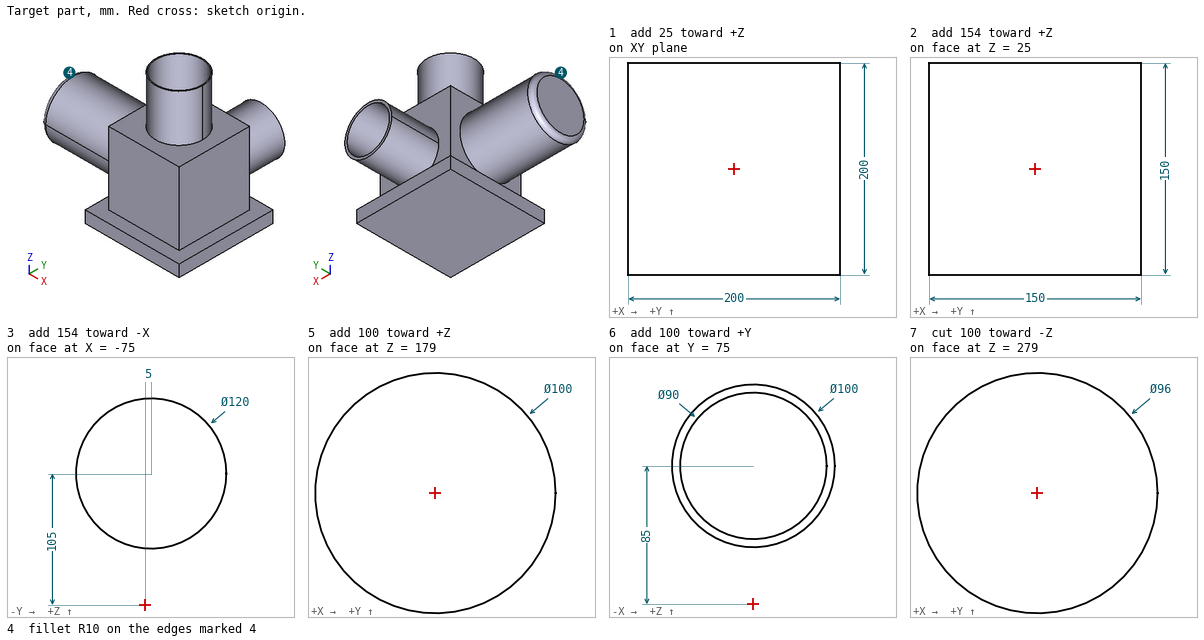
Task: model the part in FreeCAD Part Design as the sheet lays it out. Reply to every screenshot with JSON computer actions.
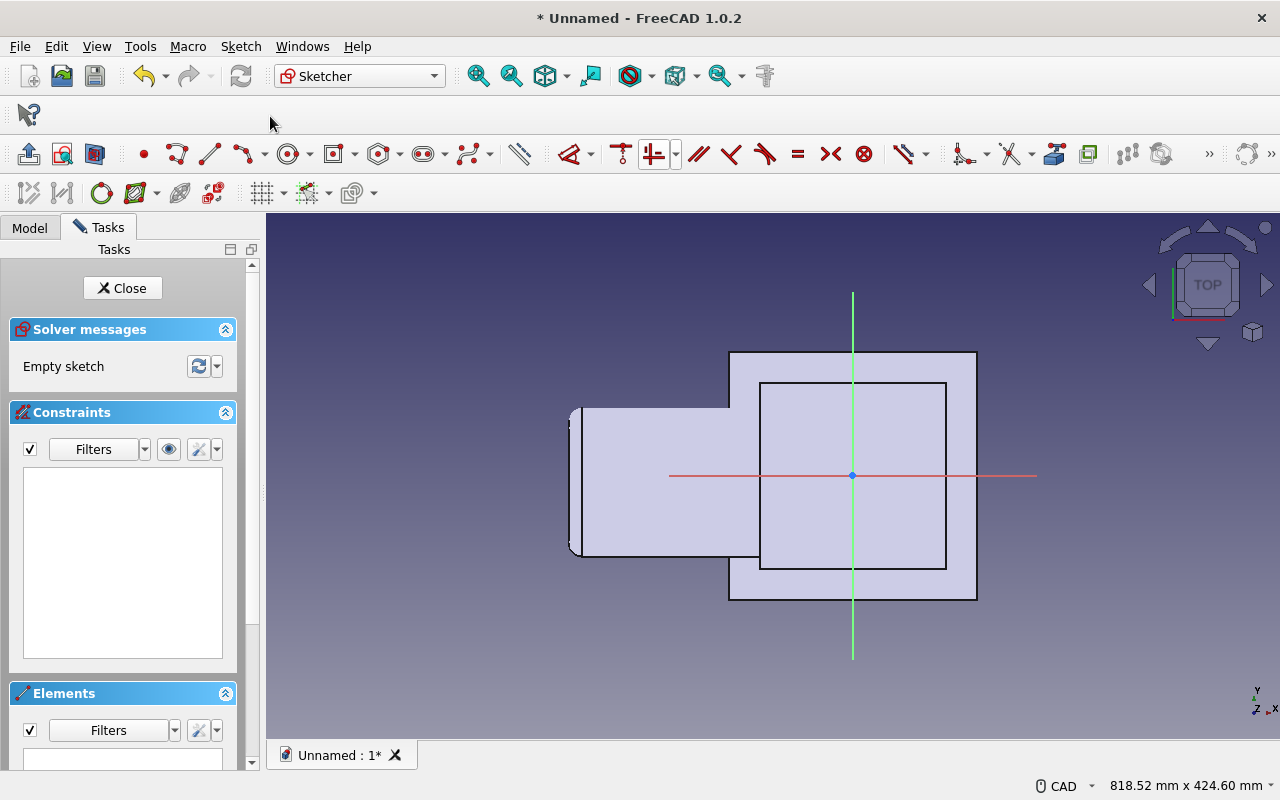
{"action": "scroll", "coordinate": [939, 476], "scroll_direction": "up", "scroll_amount": 5}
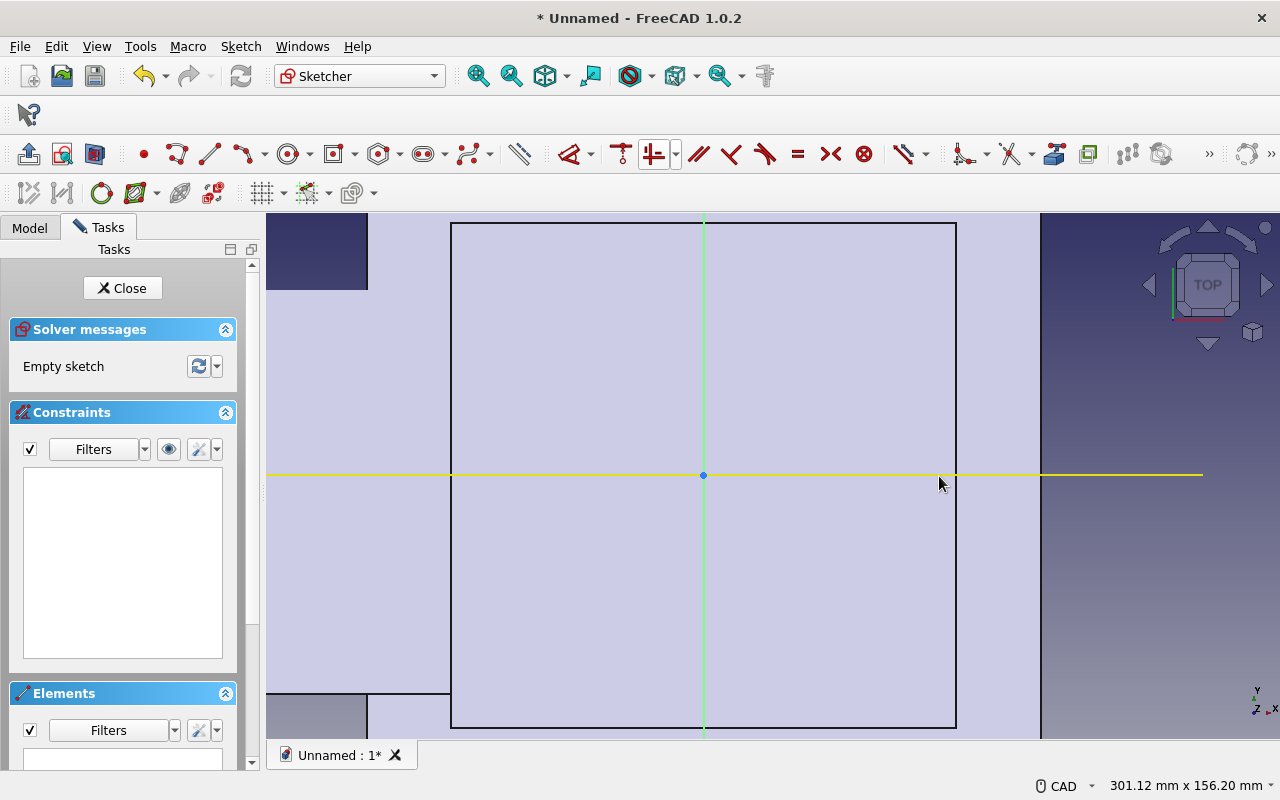
{"action": "left_click", "coordinate": [288, 154]}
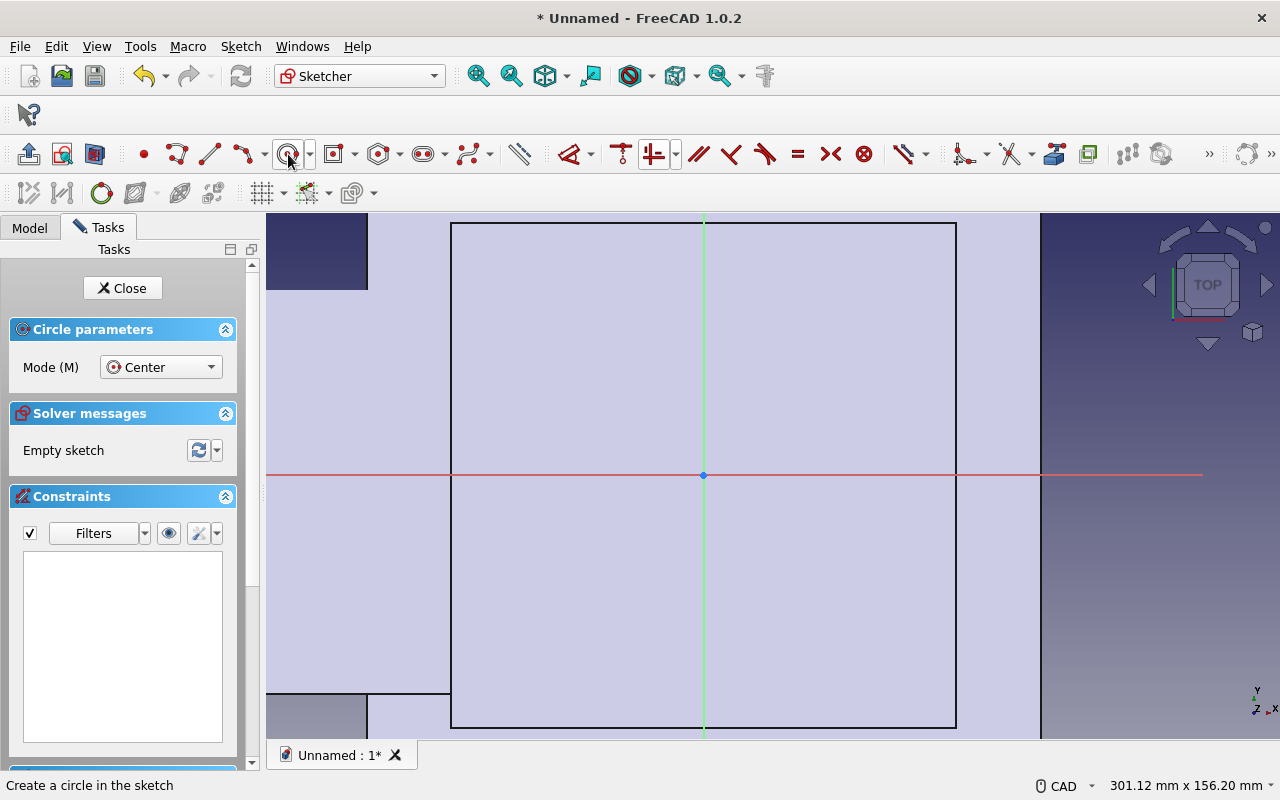
{"action": "left_click", "coordinate": [704, 475]}
{"action": "mouse_move", "coordinate": [823, 356]}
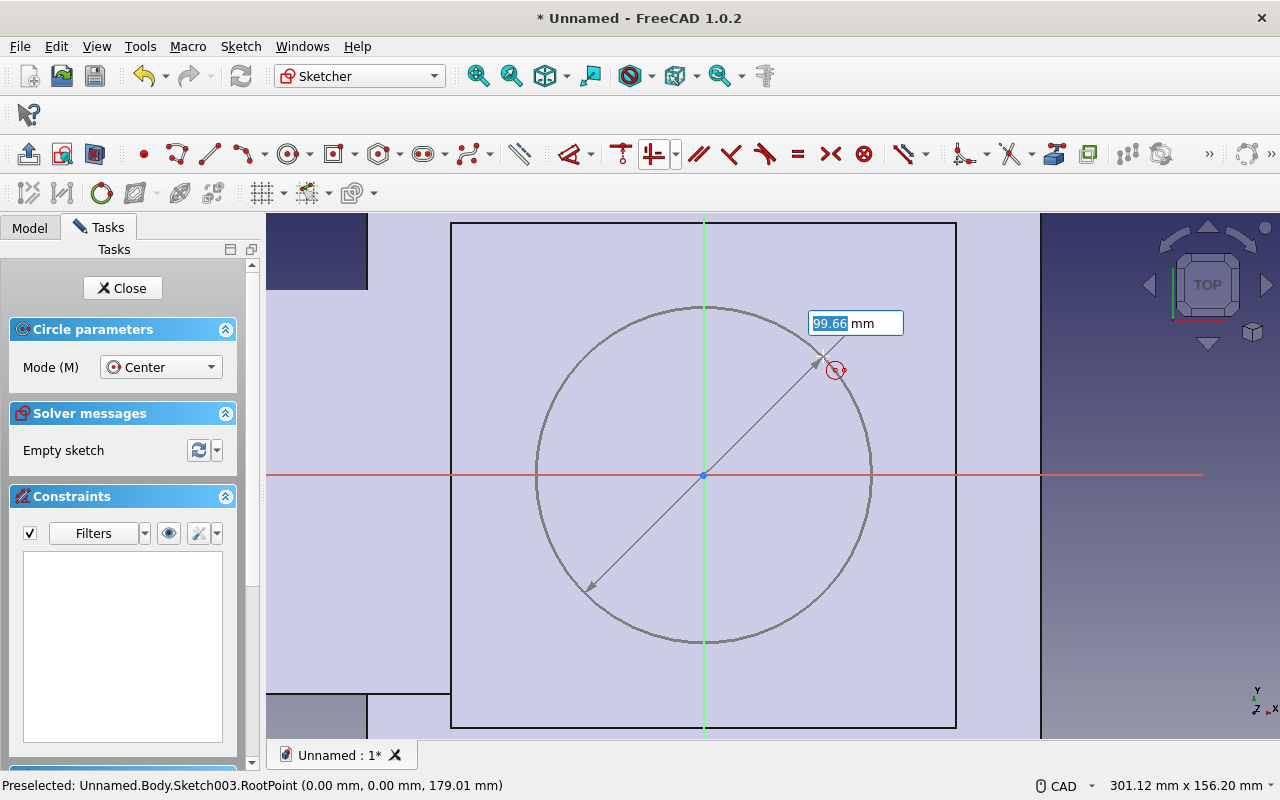
{"action": "type", "text": "100"}
{"action": "key", "text": "Return"}
{"action": "key", "text": "Escape"}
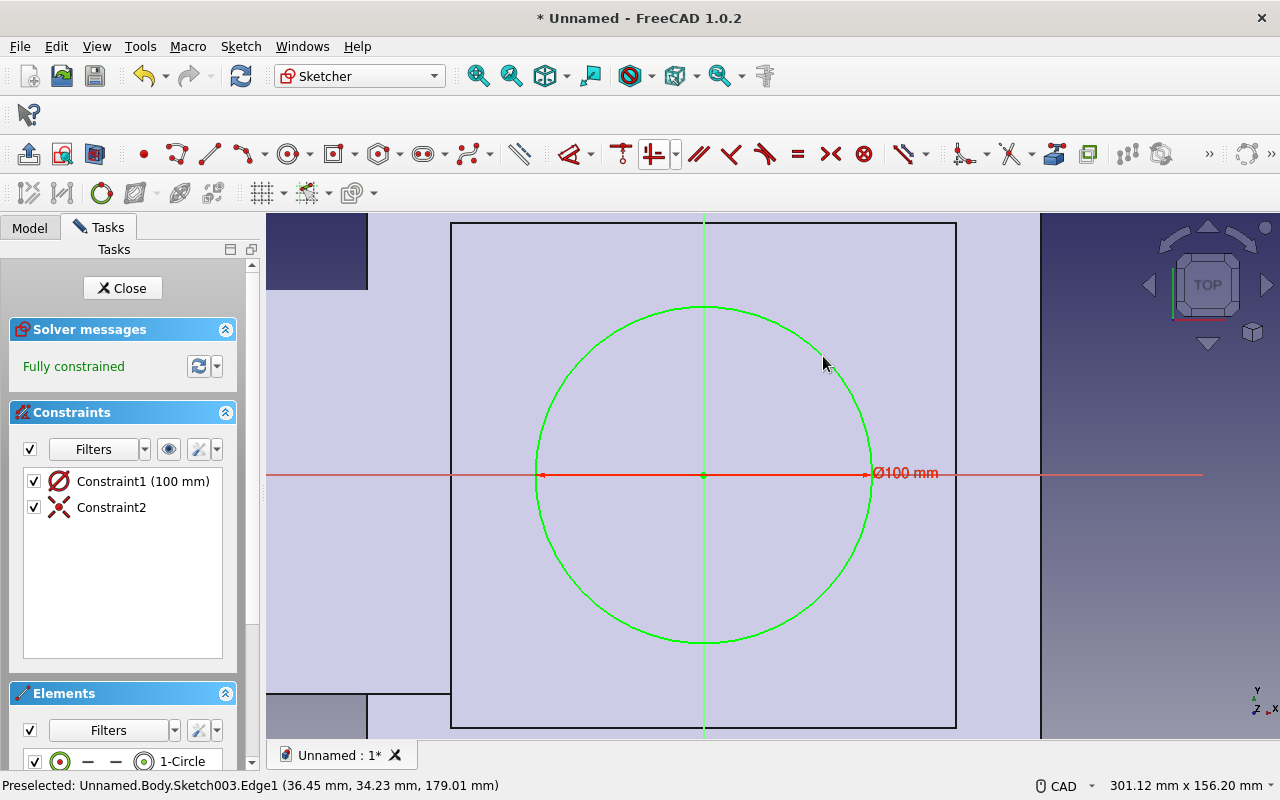
{"action": "left_click", "coordinate": [123, 288]}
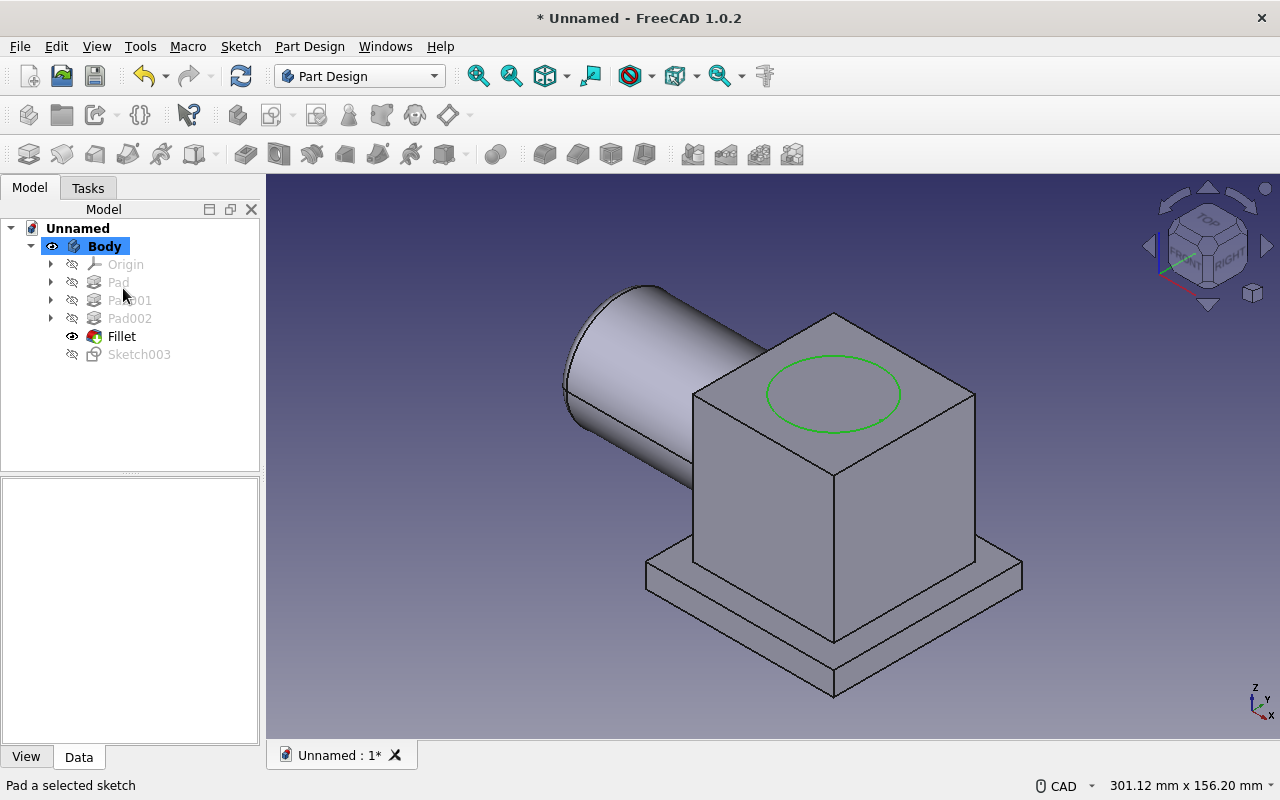
{"action": "left_click", "coordinate": [29, 154]}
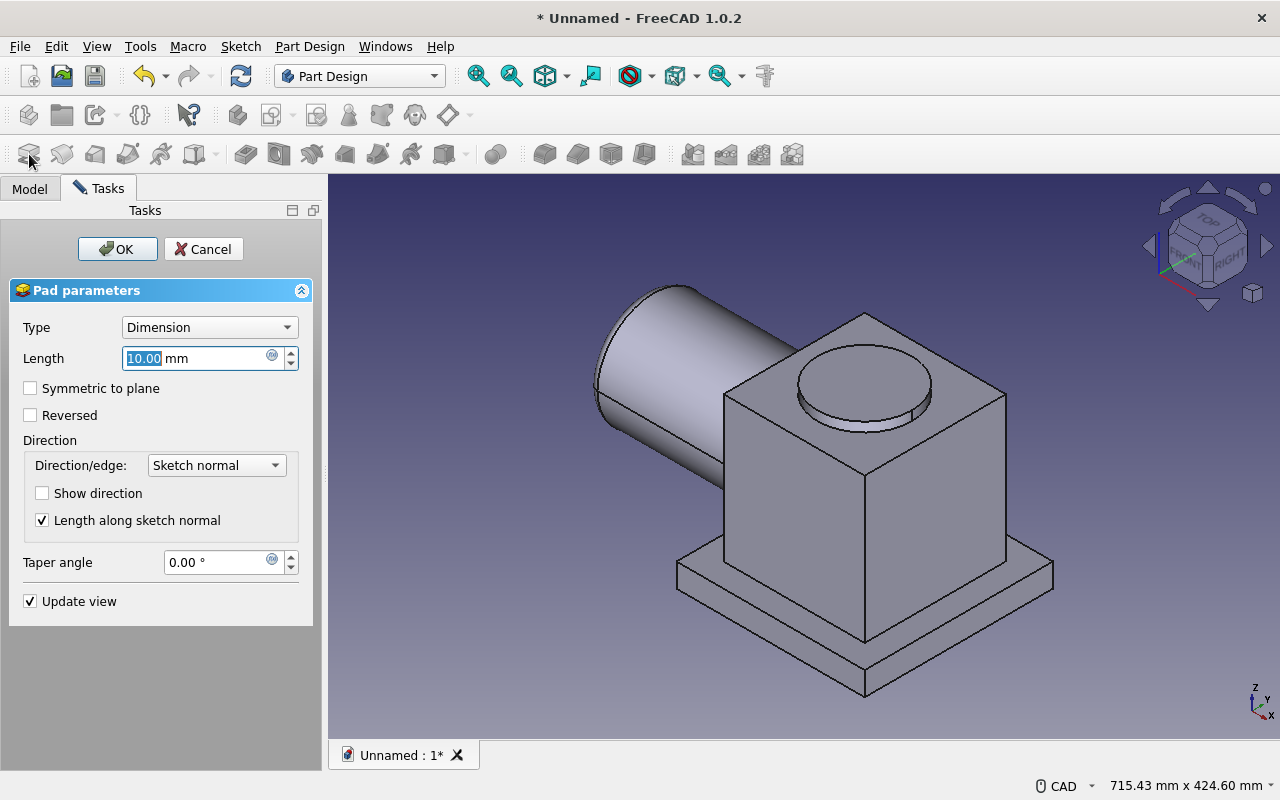
{"action": "type", "text": "100"}
{"action": "key", "text": "Tab"}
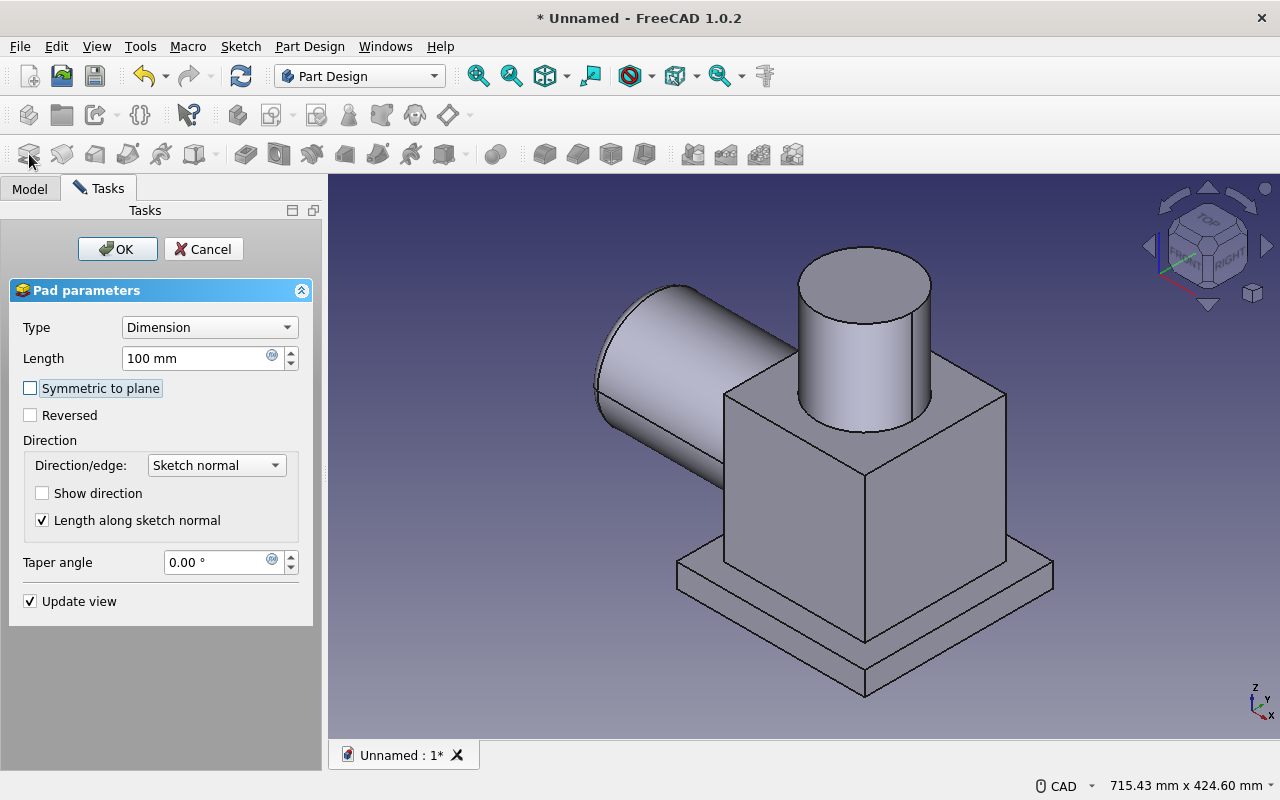
{"action": "left_click", "coordinate": [118, 249]}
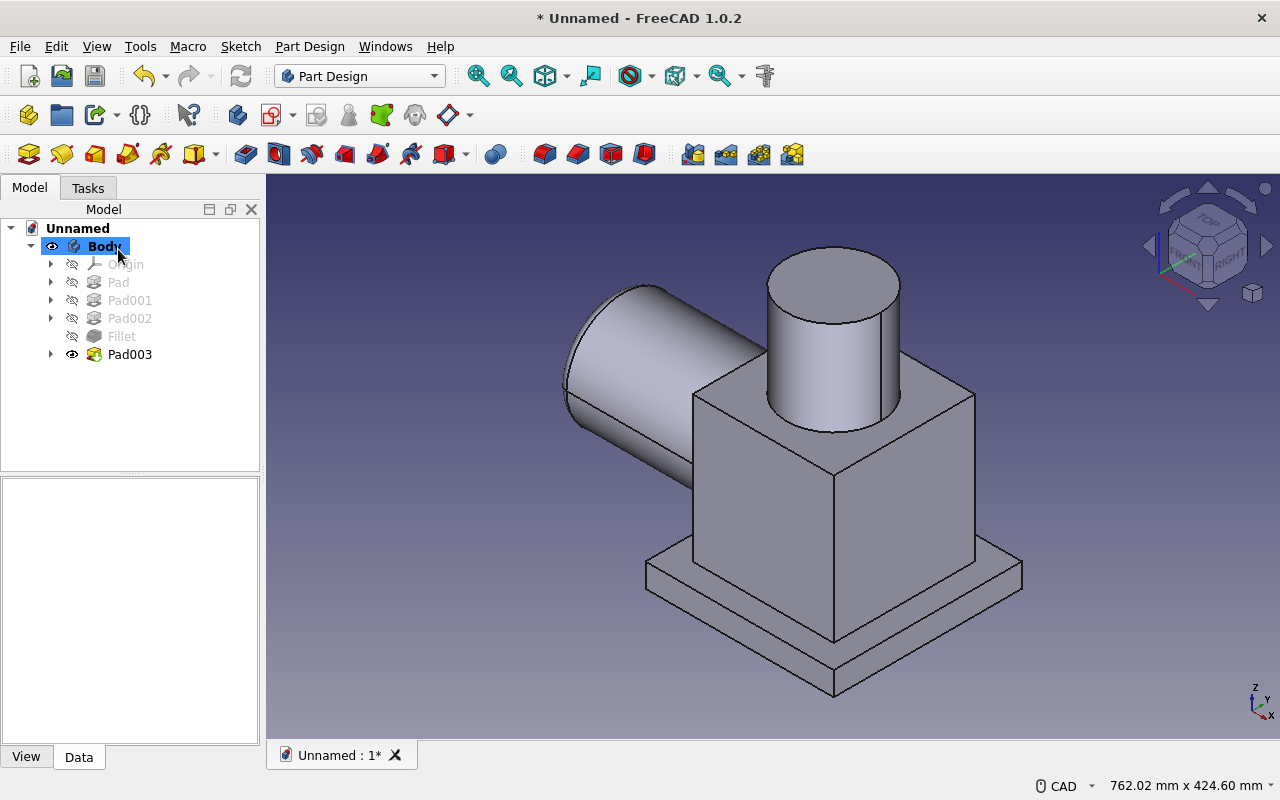
{"action": "left_click", "coordinate": [479, 76]}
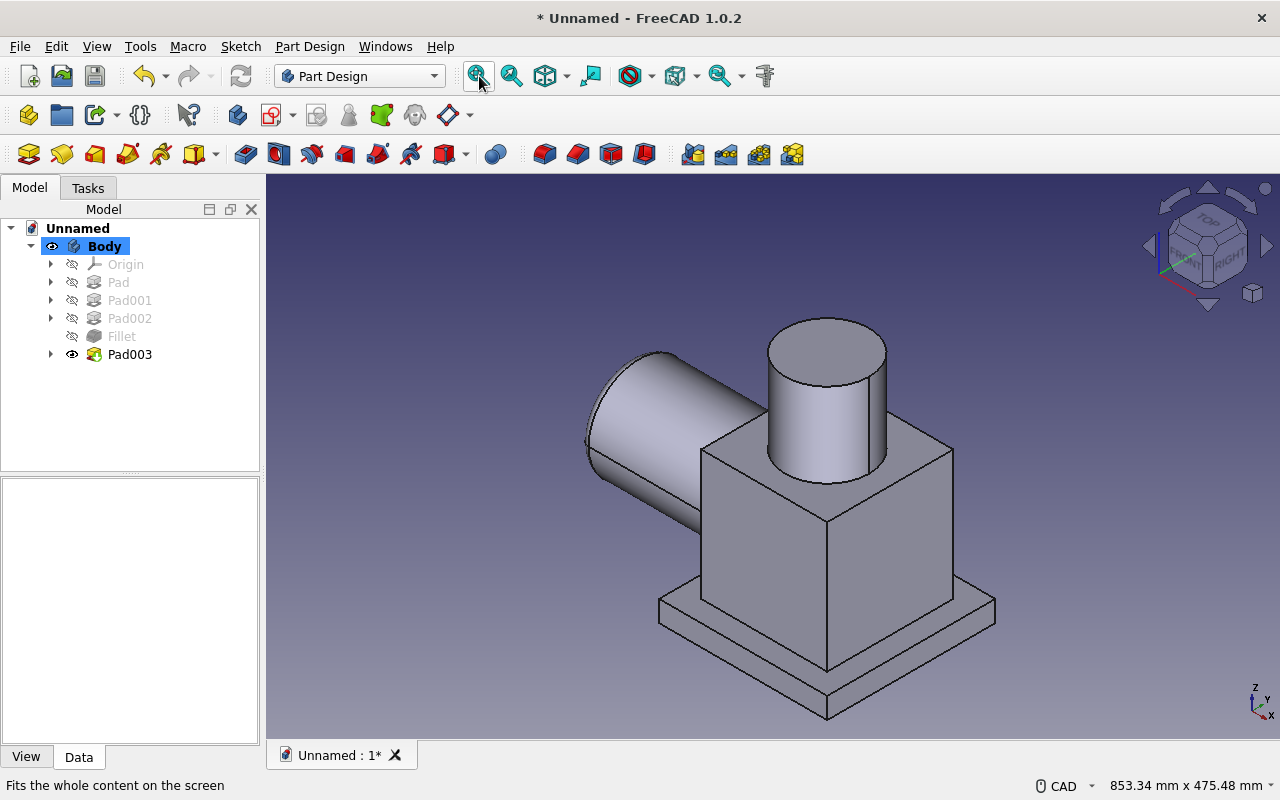
{"action": "key", "text": "4"}